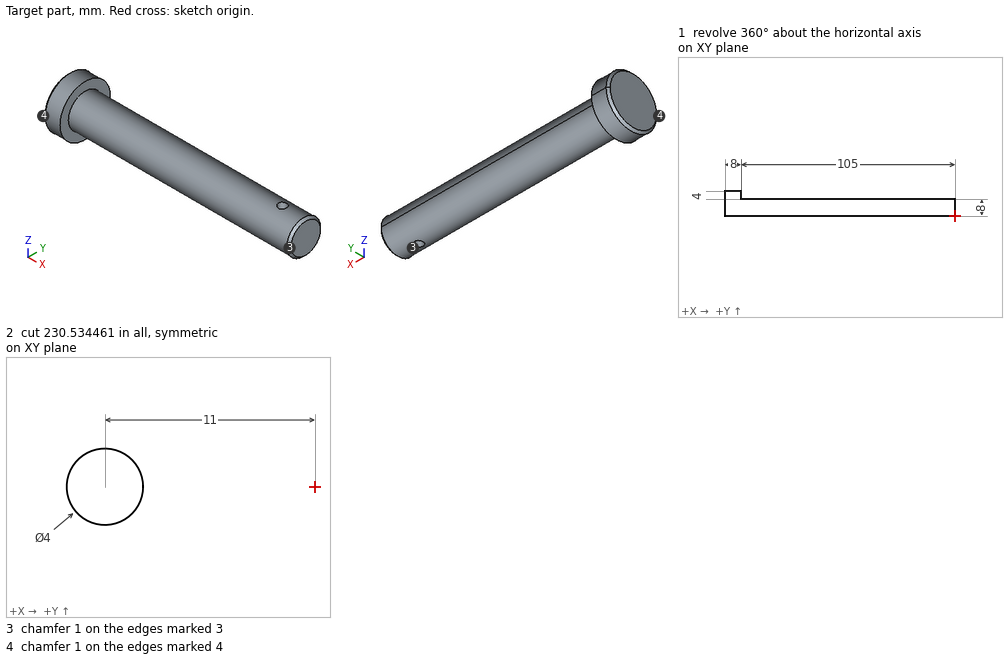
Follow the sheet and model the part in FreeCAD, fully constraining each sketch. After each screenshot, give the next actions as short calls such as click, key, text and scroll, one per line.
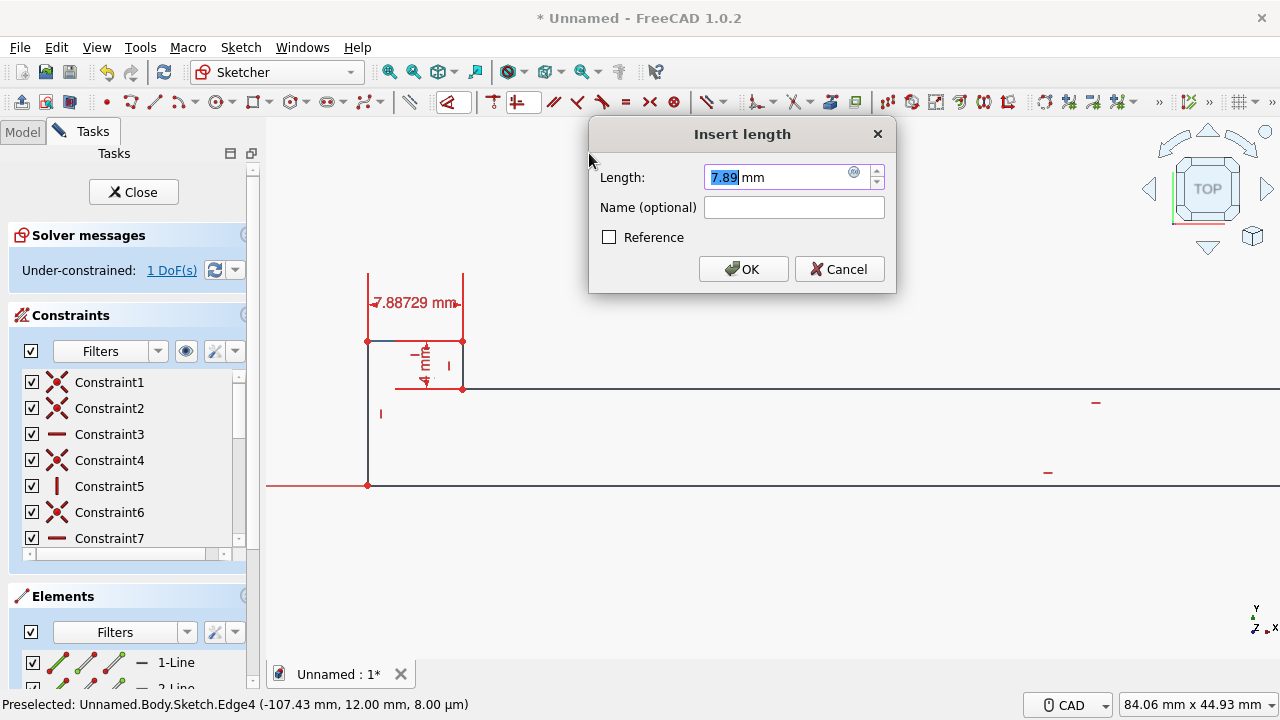
text(8)
key(Return)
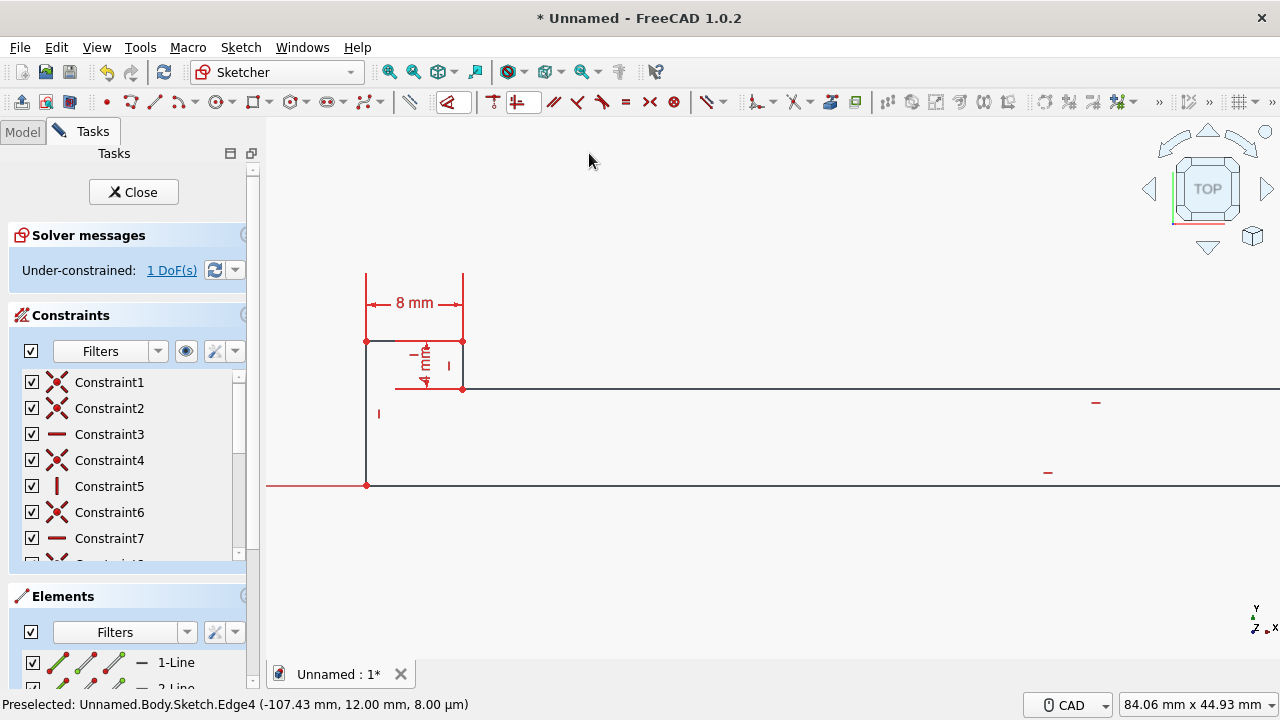
click(843, 389)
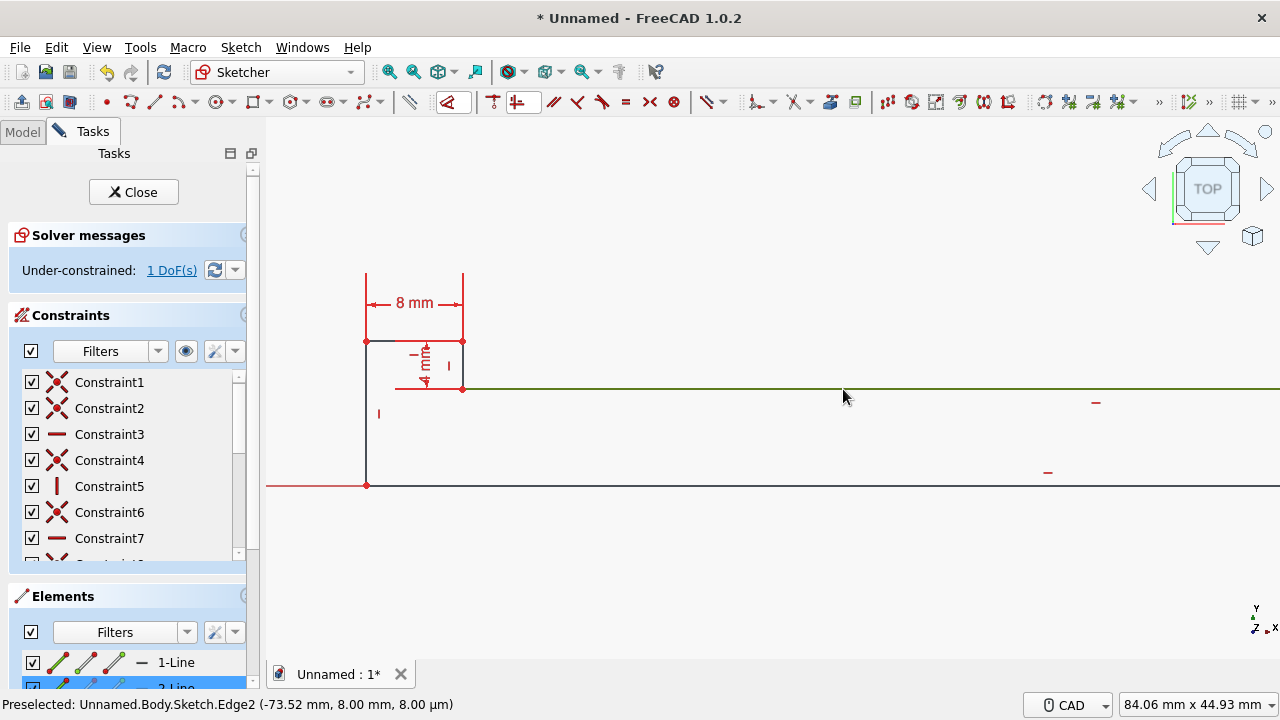
click(466, 102)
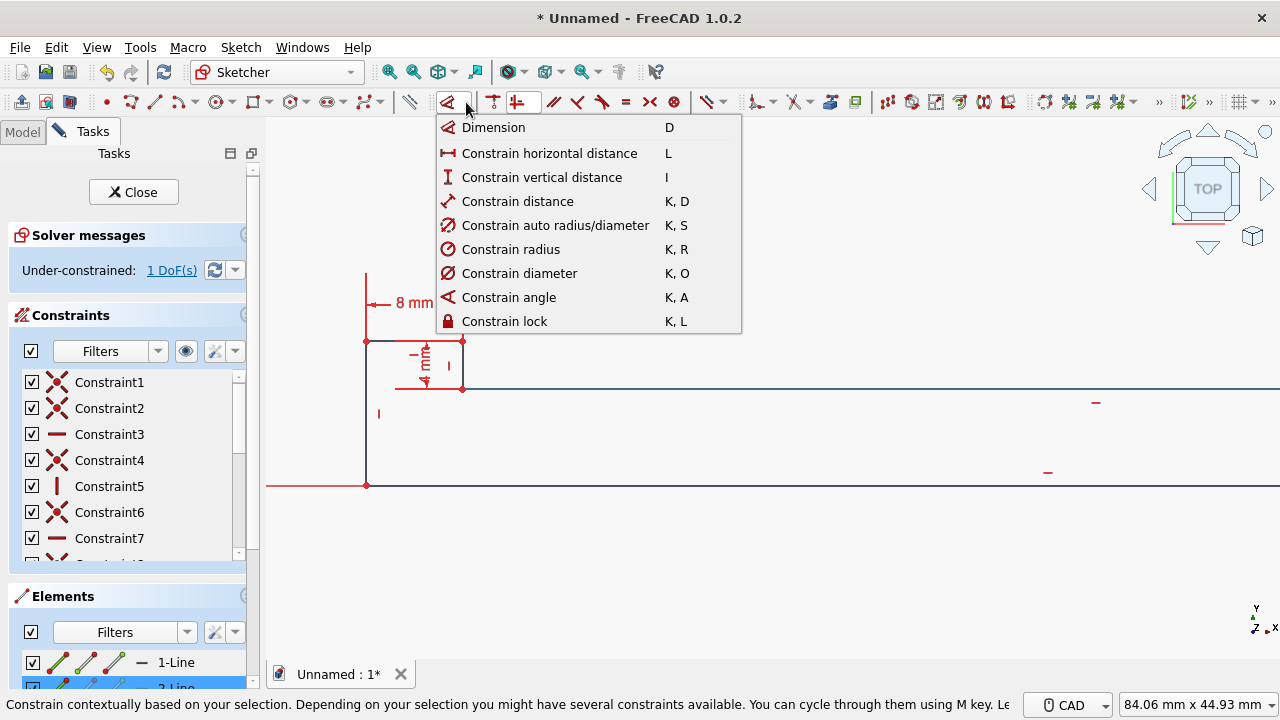
click(589, 153)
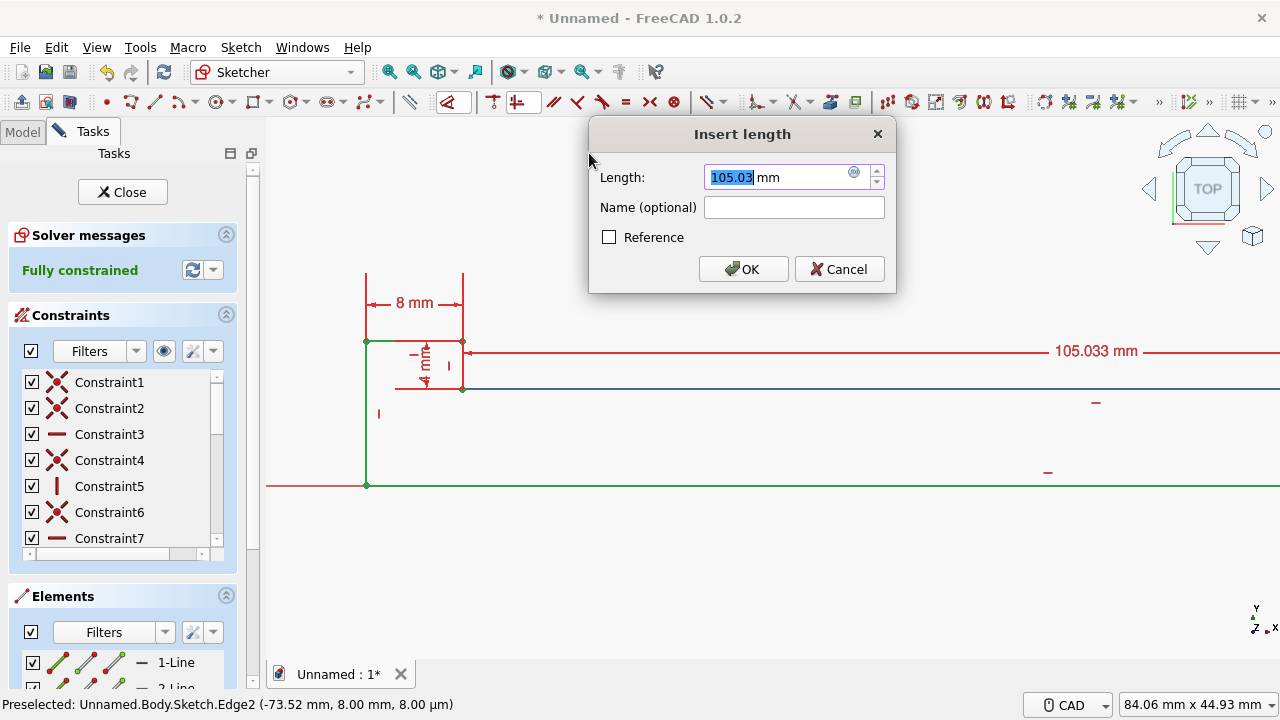
text(105)
key(Return)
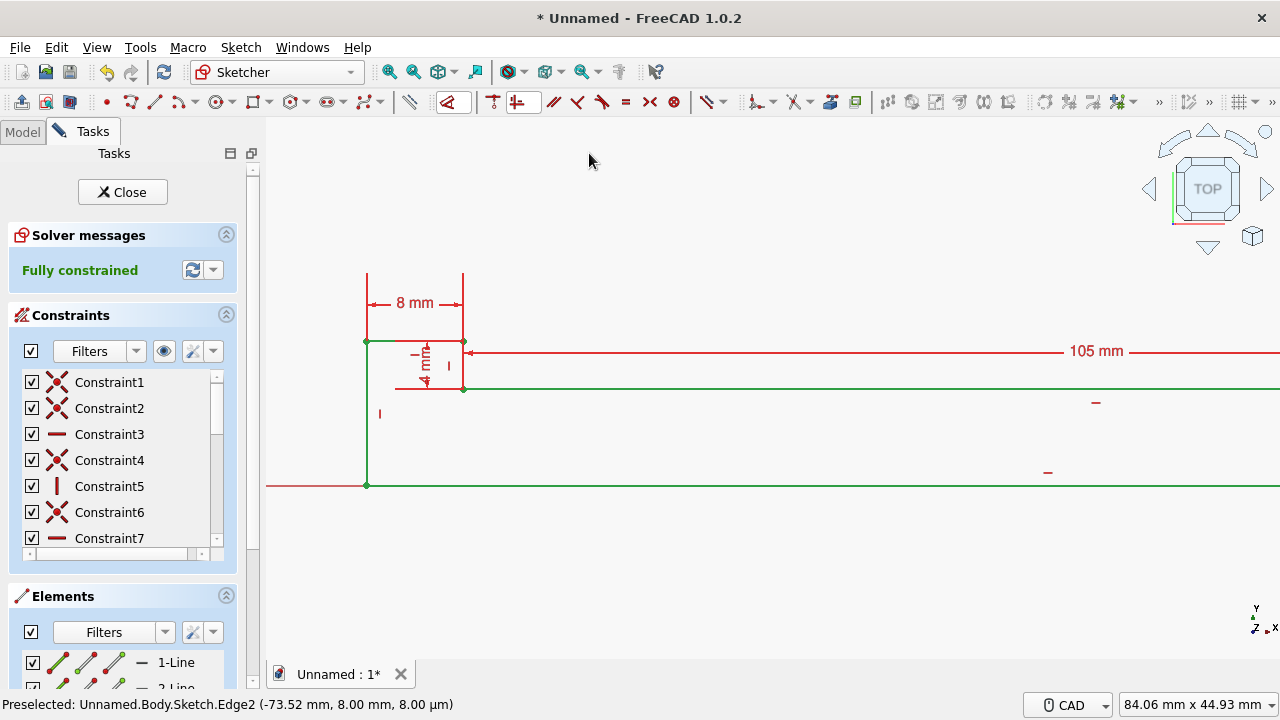
click(123, 192)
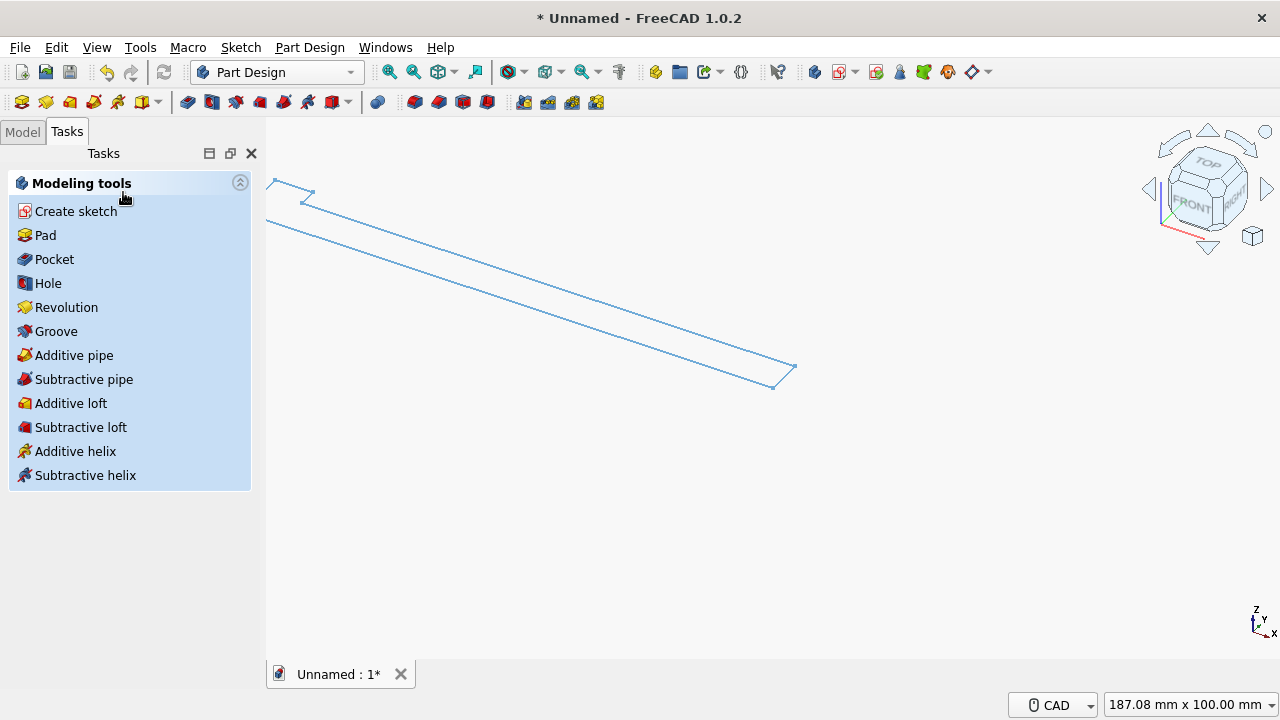
click(46, 102)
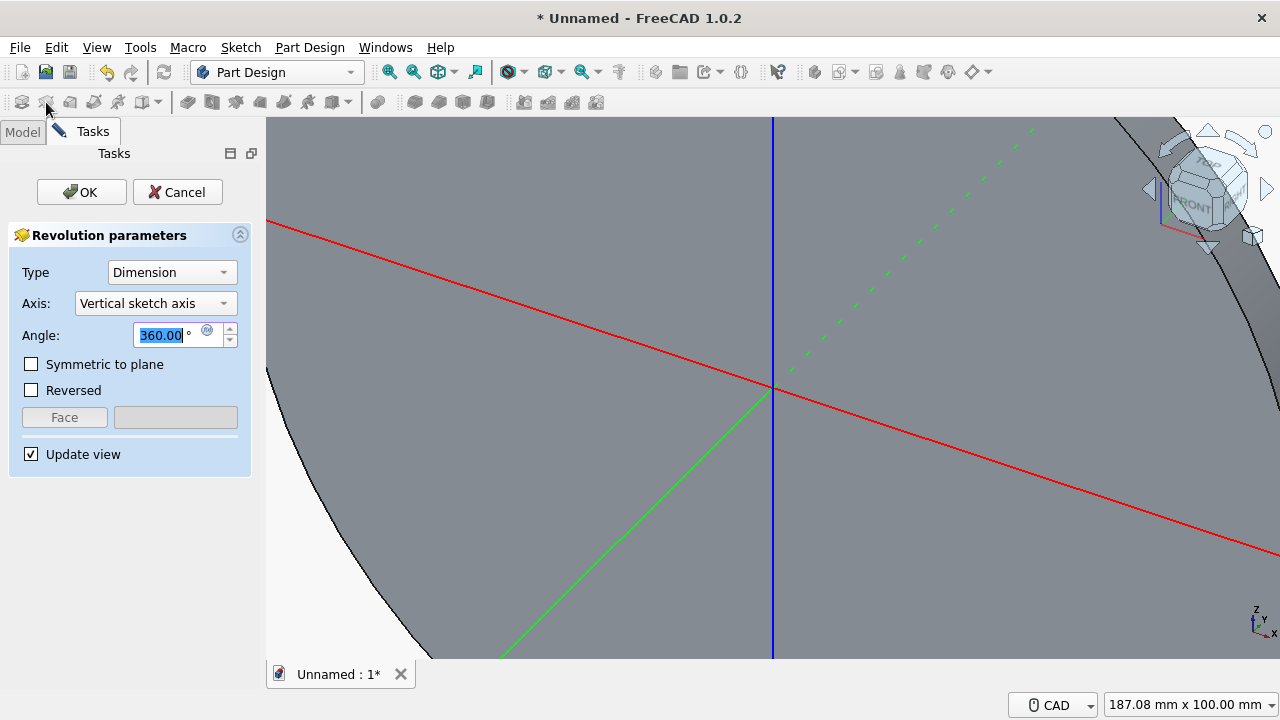
click(156, 304)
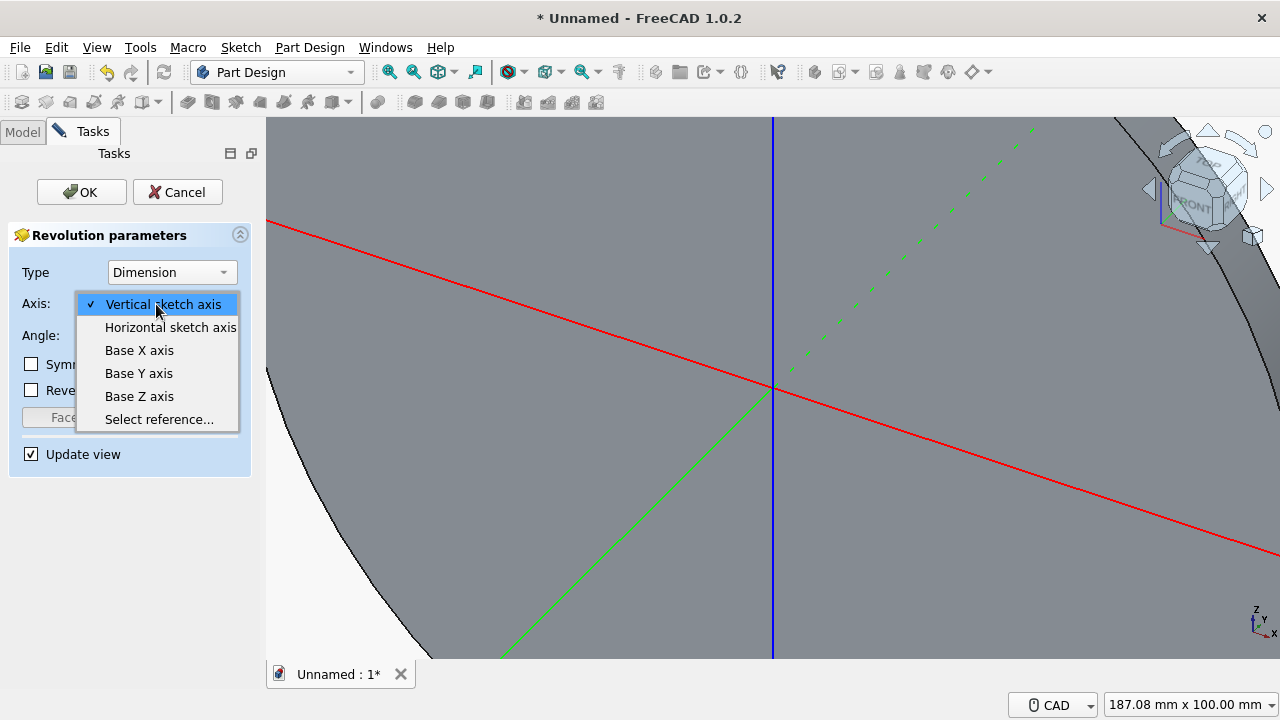
click(156, 328)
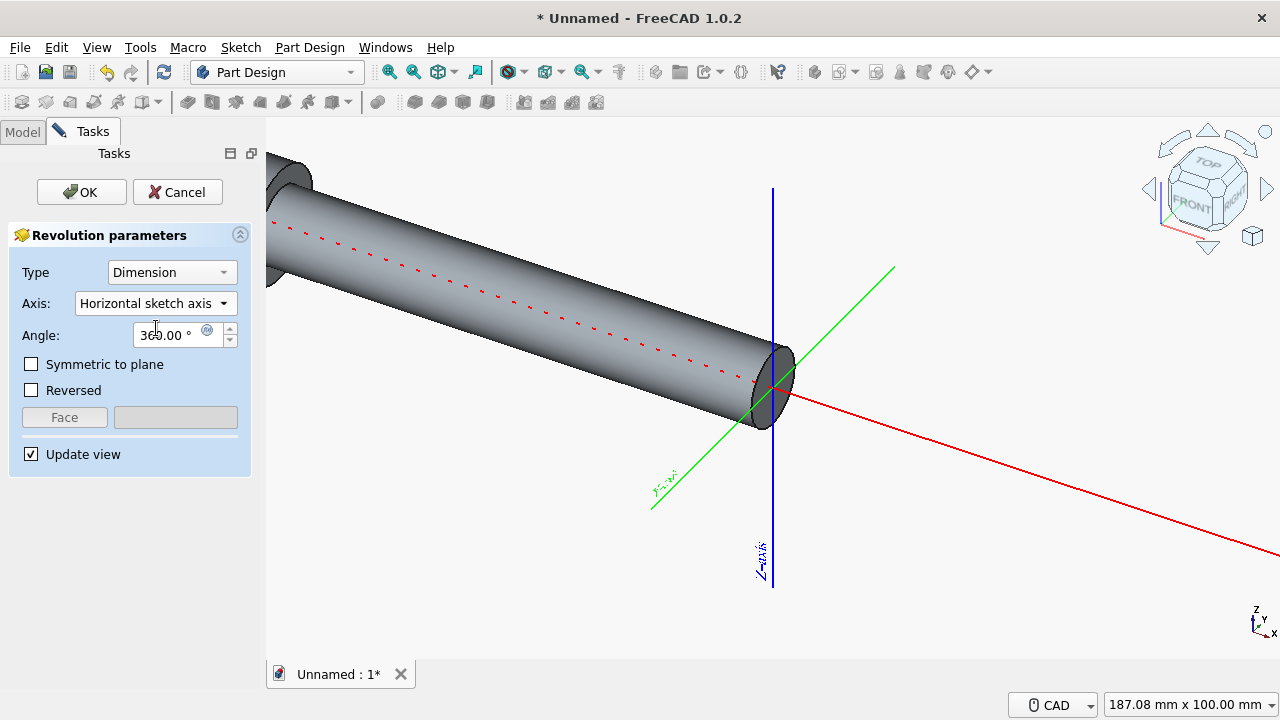
click(82, 192)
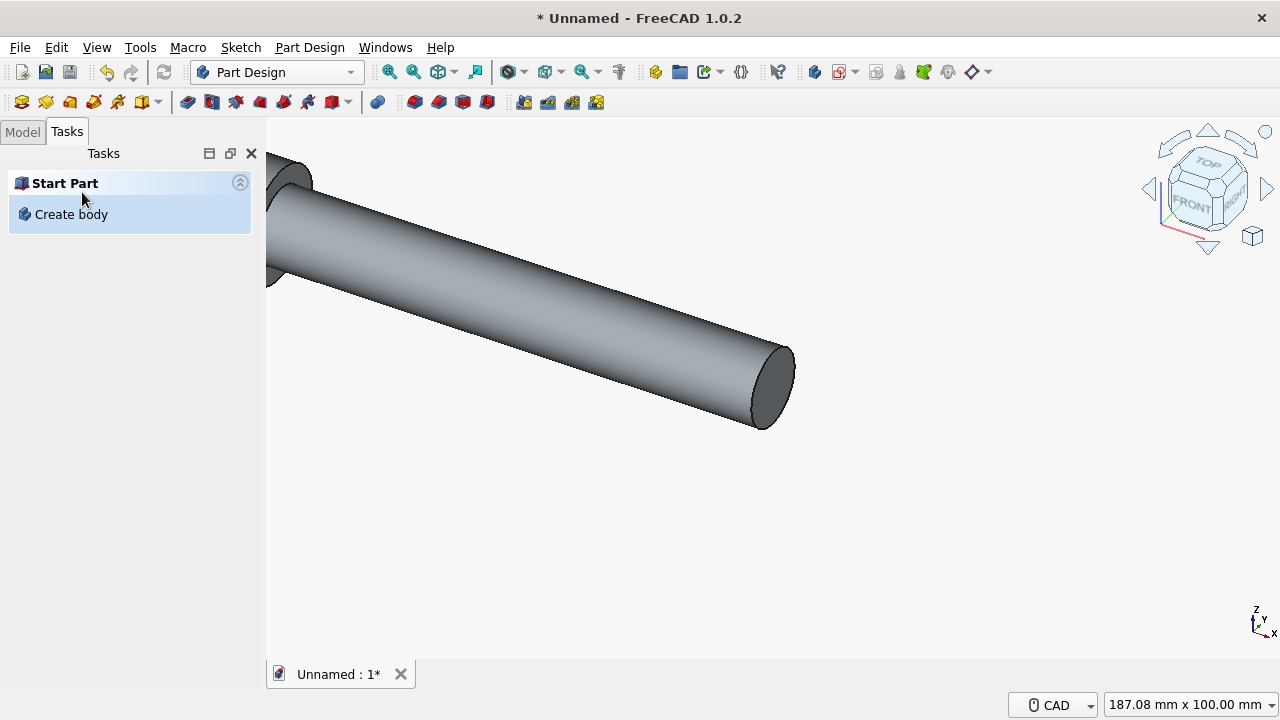
click(390, 72)